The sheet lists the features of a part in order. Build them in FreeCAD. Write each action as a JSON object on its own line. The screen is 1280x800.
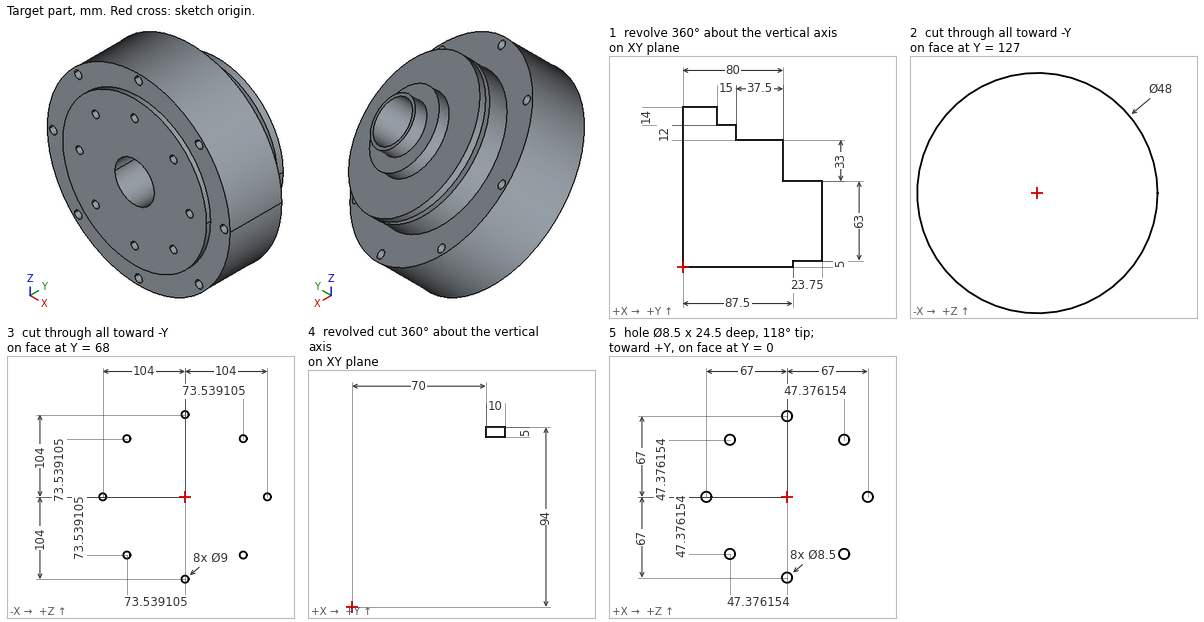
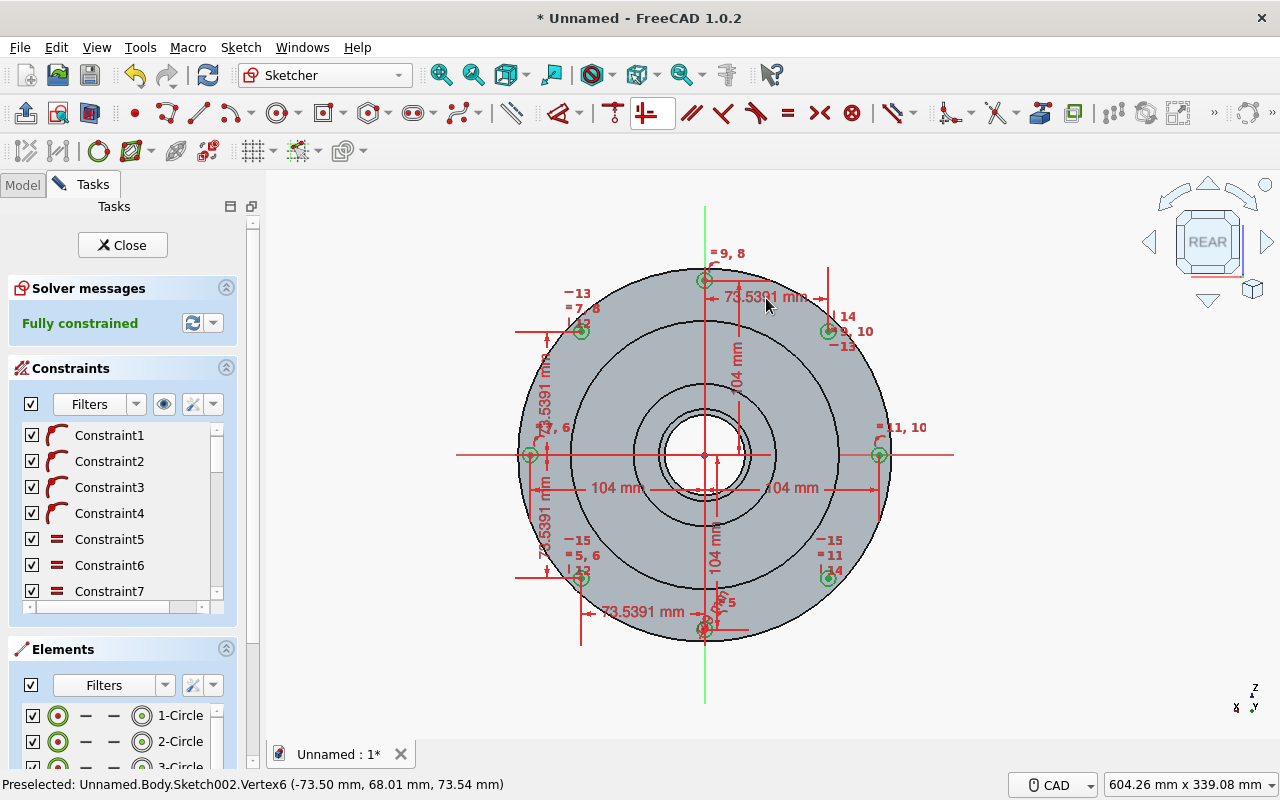
{"action": "left_click", "coordinate": [123, 245]}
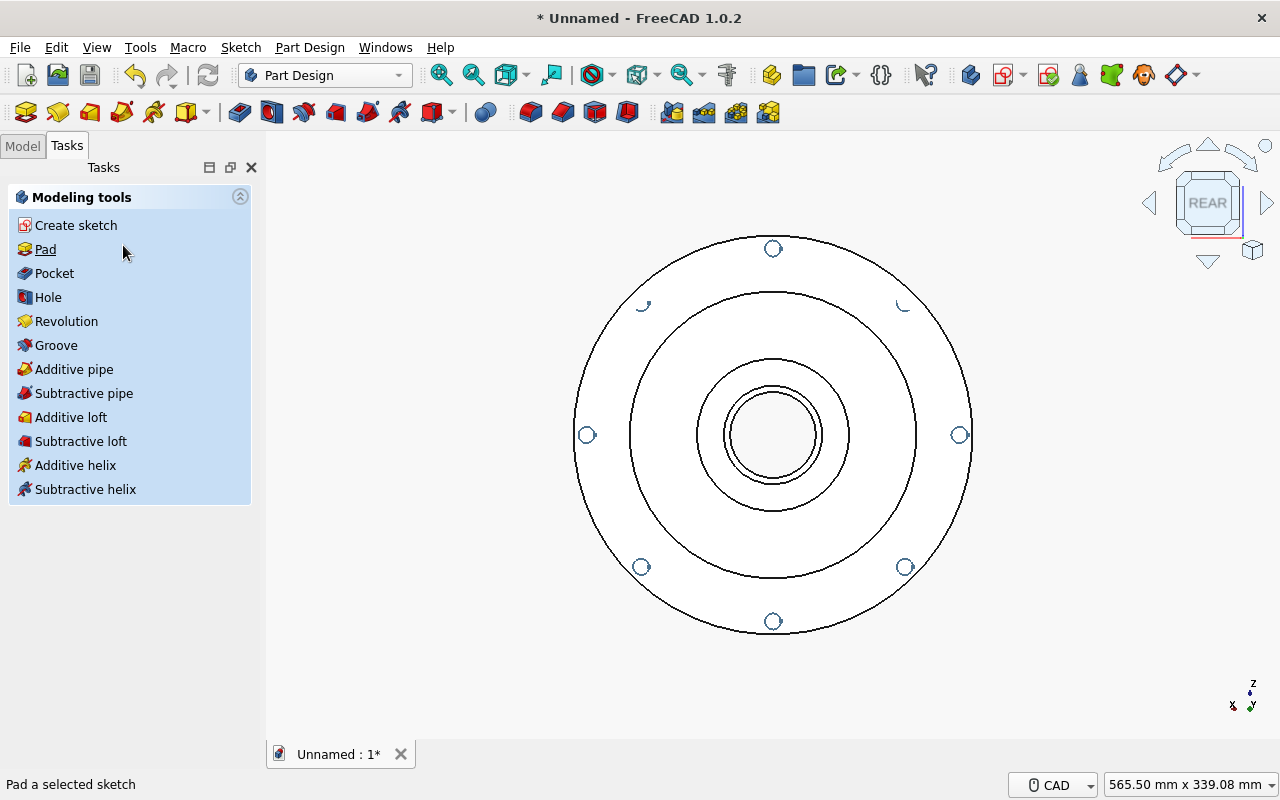
{"action": "left_click", "coordinate": [240, 112]}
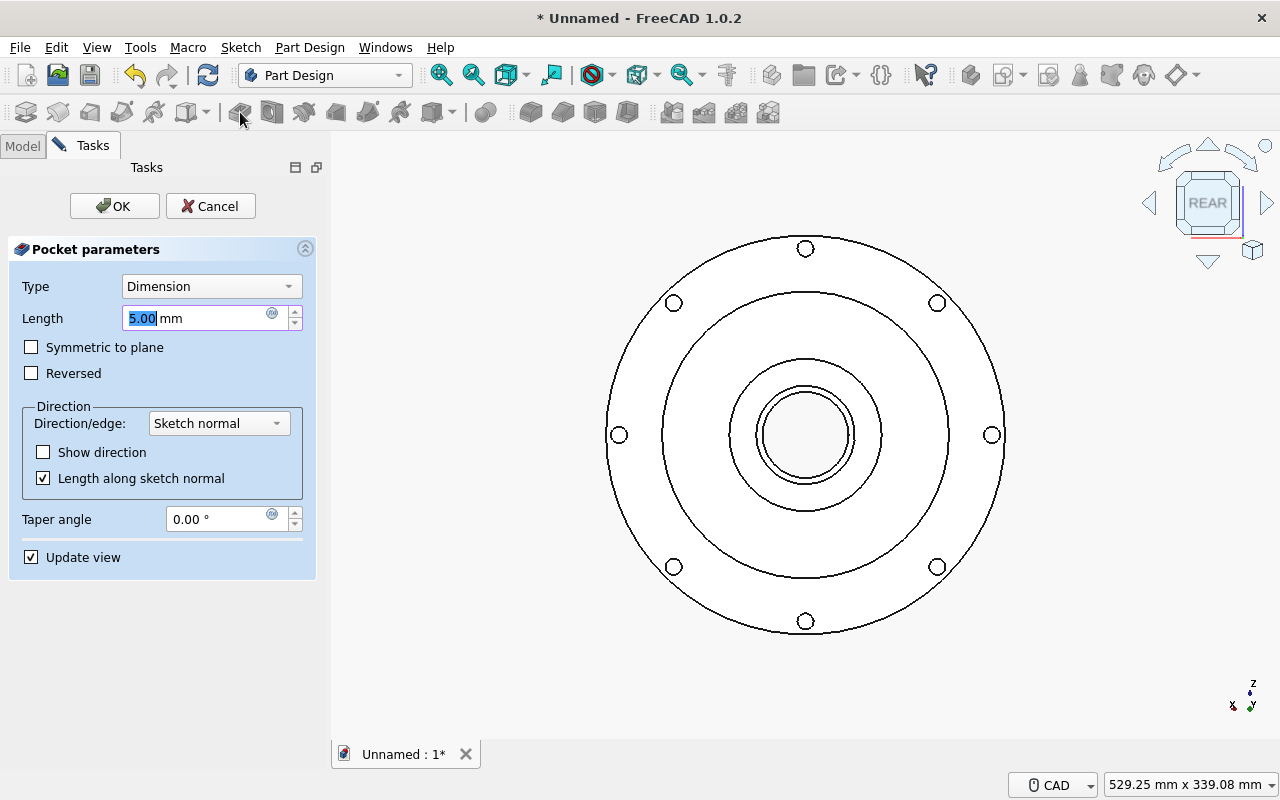
{"action": "left_click", "coordinate": [212, 286]}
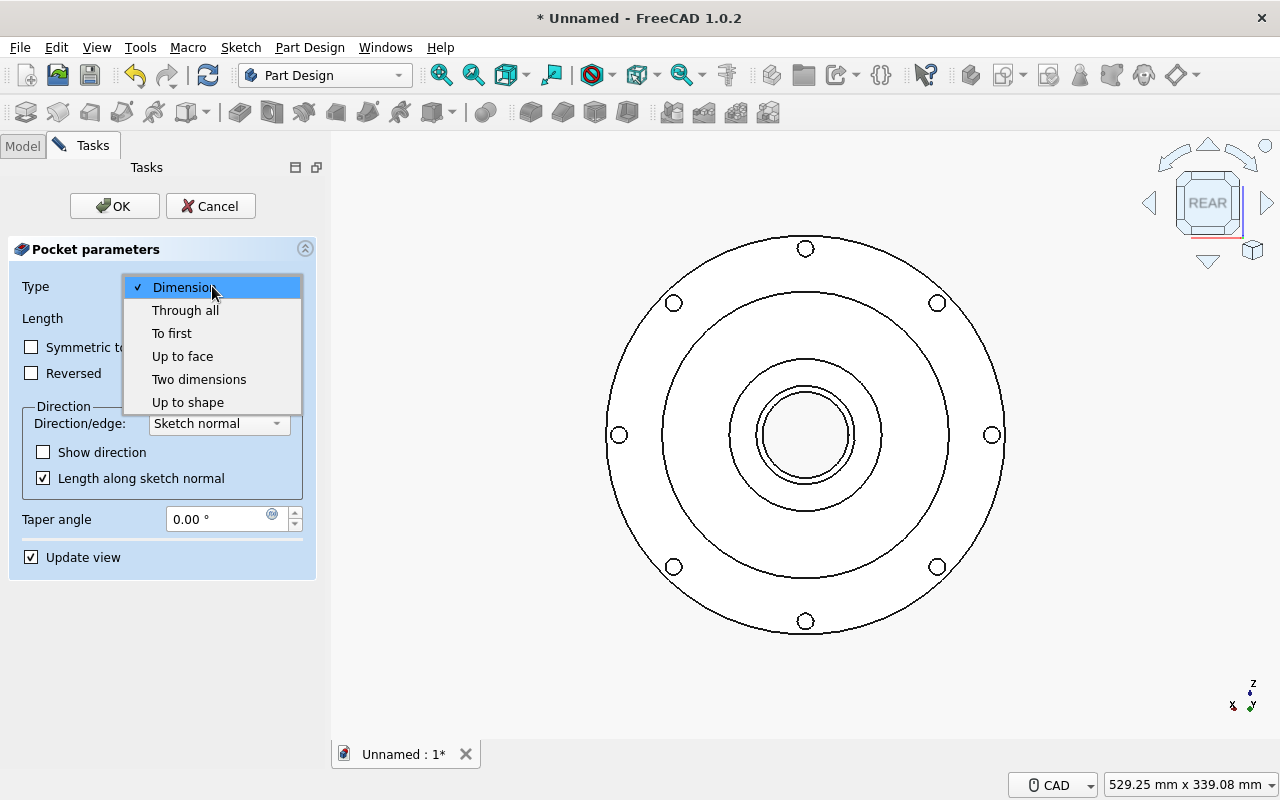
{"action": "left_click", "coordinate": [212, 310]}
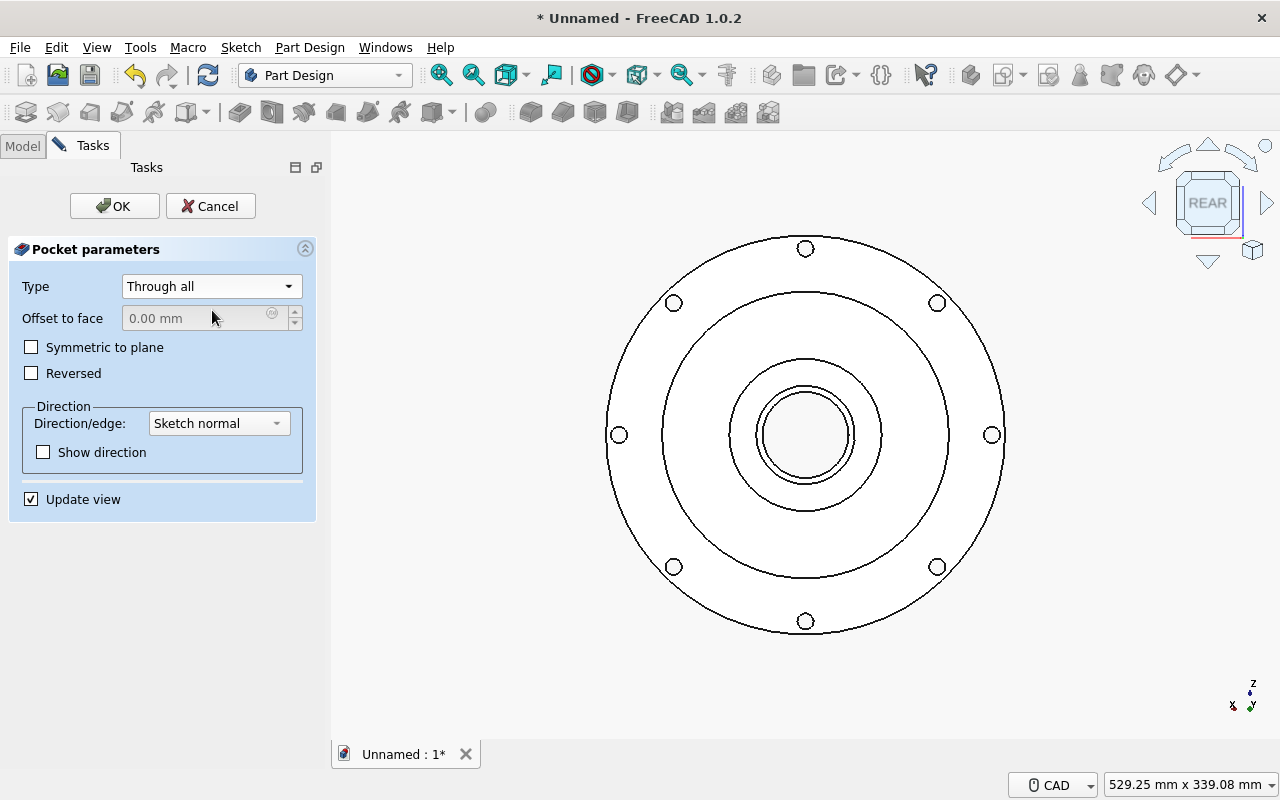
{"action": "left_click", "coordinate": [115, 206]}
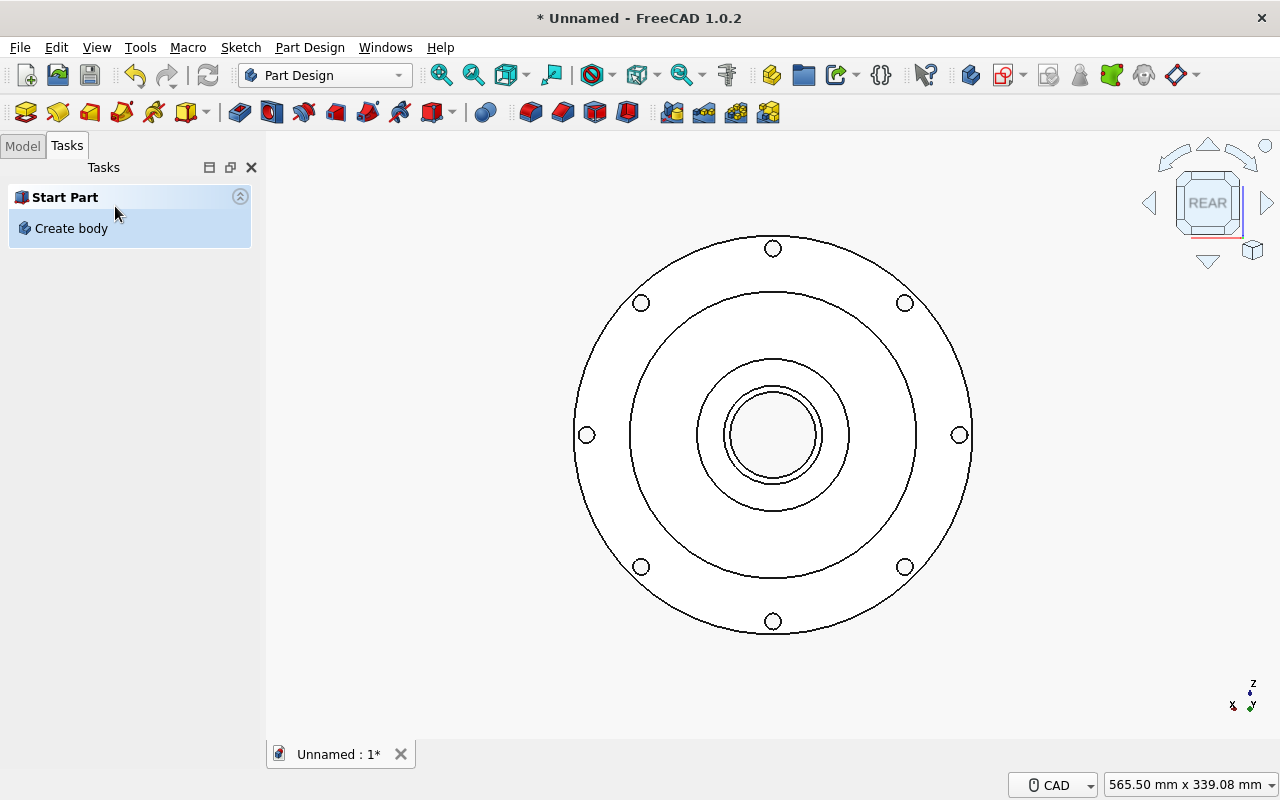
{"action": "left_click", "coordinate": [1004, 76]}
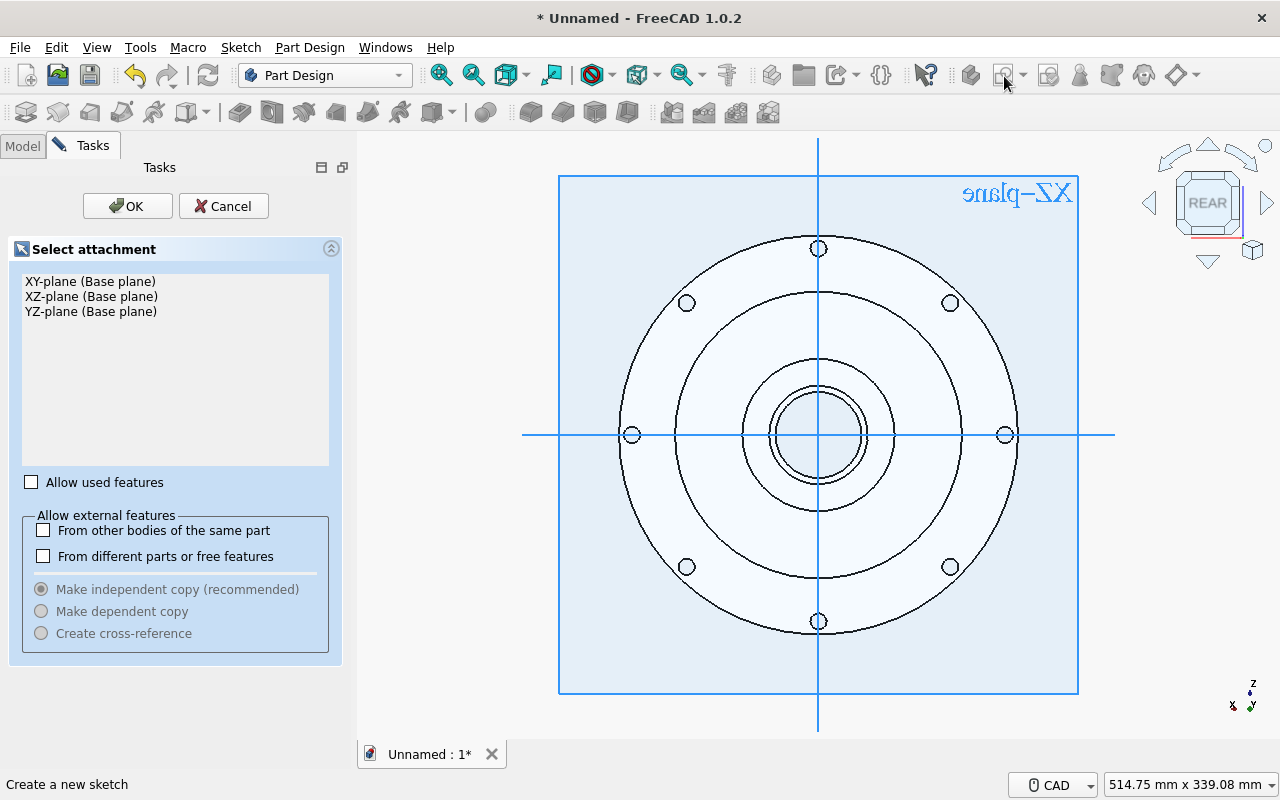
{"action": "left_click", "coordinate": [82, 282]}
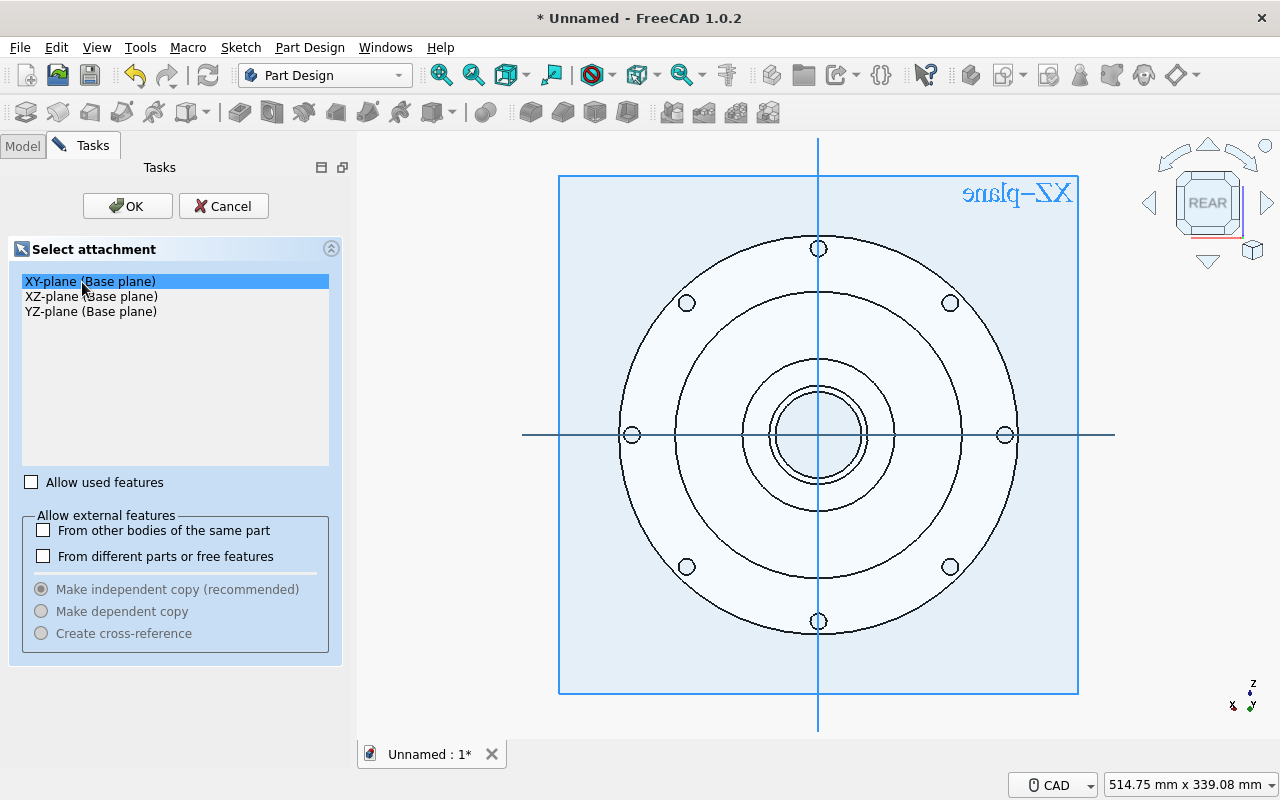
{"action": "left_click", "coordinate": [128, 206]}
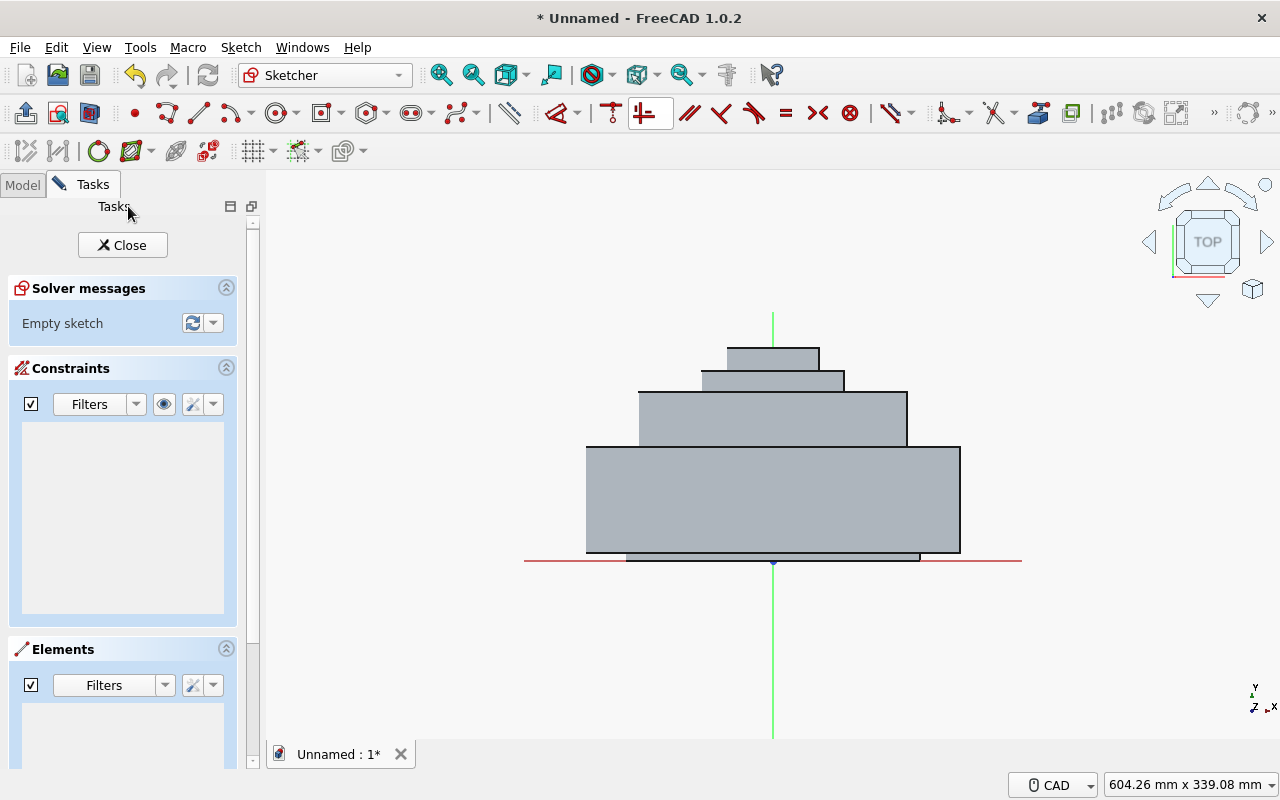
{"action": "left_click", "coordinate": [90, 114]}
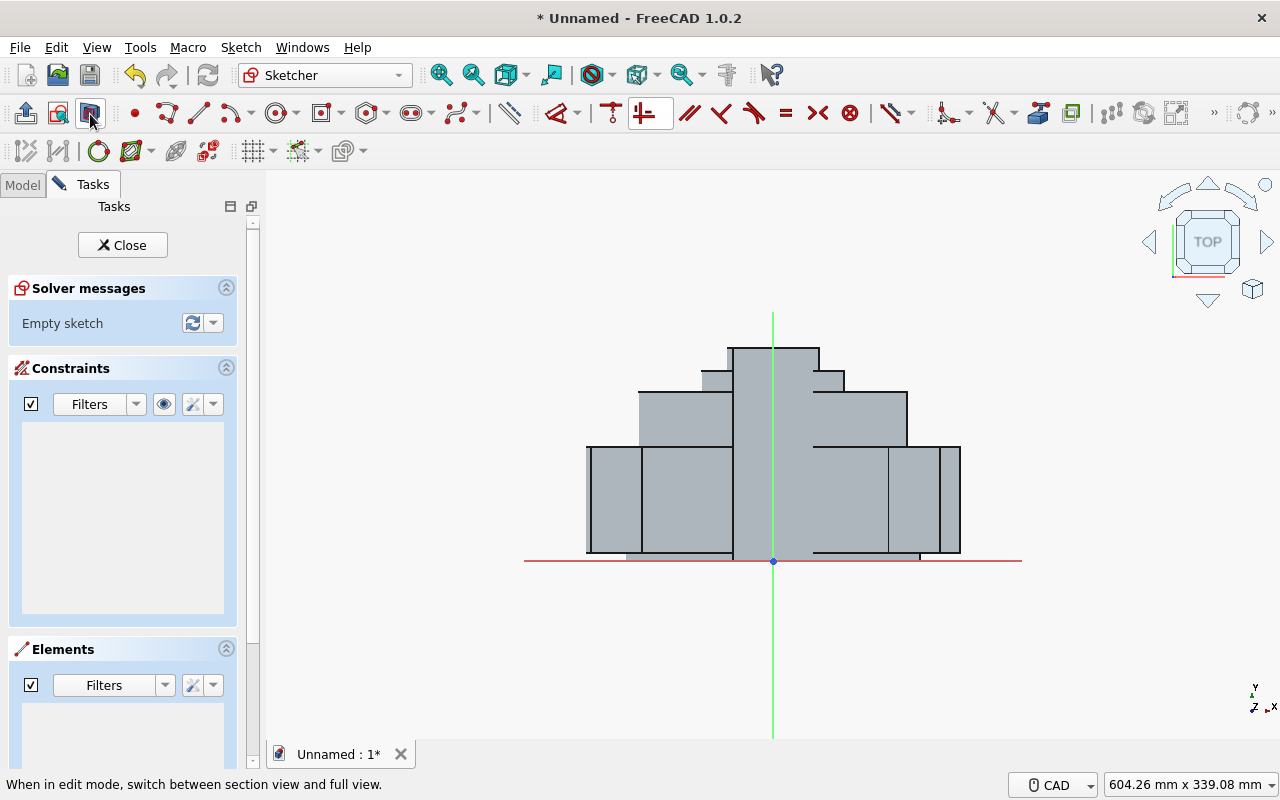
{"action": "scroll", "coordinate": [909, 405], "scroll_direction": "up", "scroll_amount": 15}